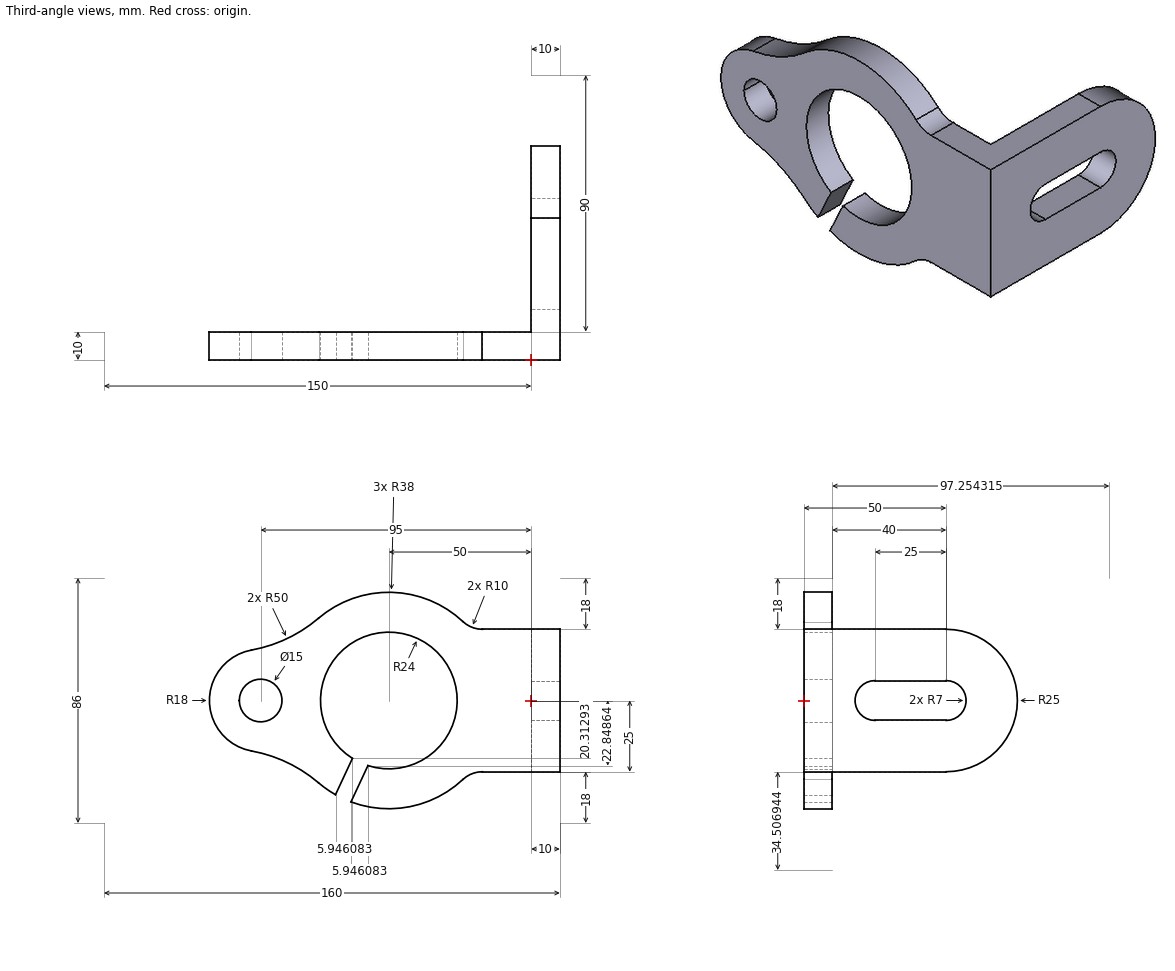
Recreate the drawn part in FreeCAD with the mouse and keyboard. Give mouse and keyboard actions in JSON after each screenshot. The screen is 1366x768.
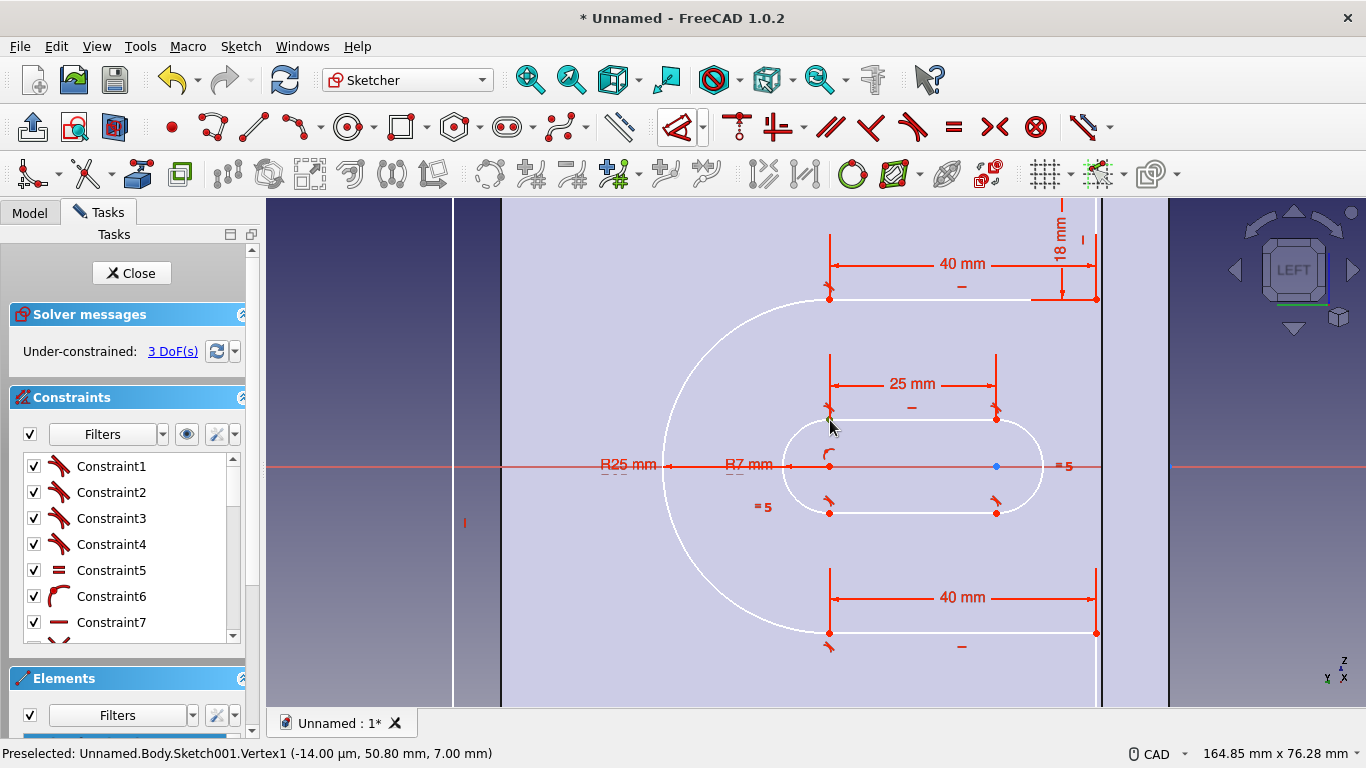
{"action": "key", "text": "l"}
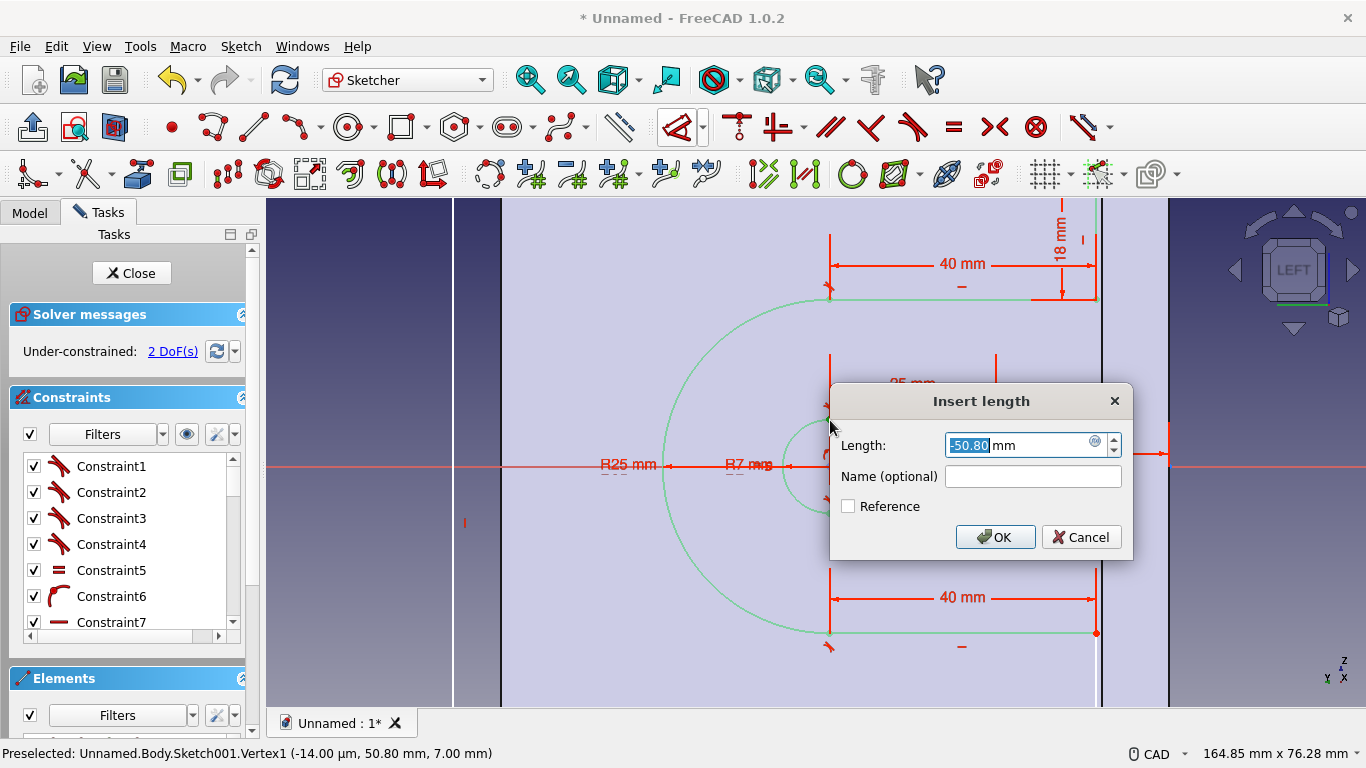
{"action": "type", "text": "-50"}
{"action": "key", "text": "Return"}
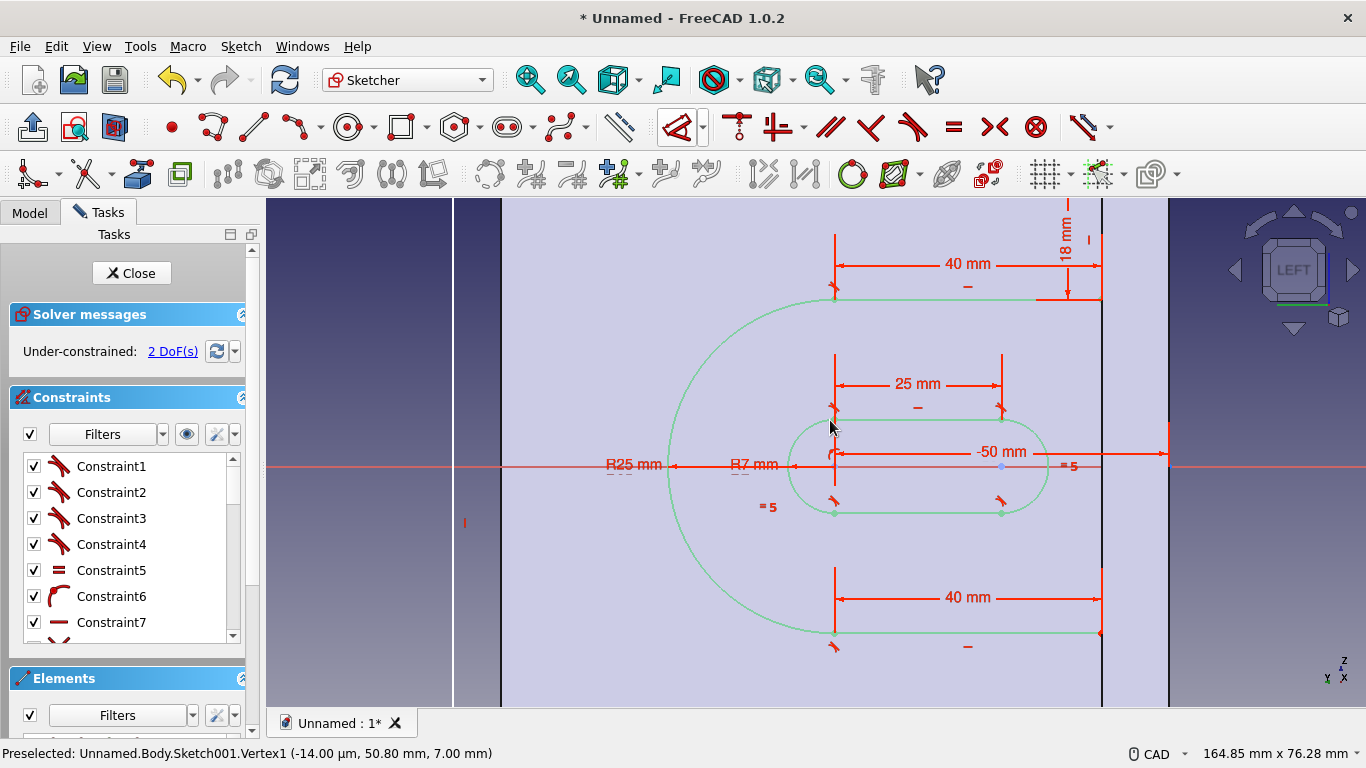
{"action": "scroll", "coordinate": [696, 396], "scroll_direction": "down", "scroll_amount": 4}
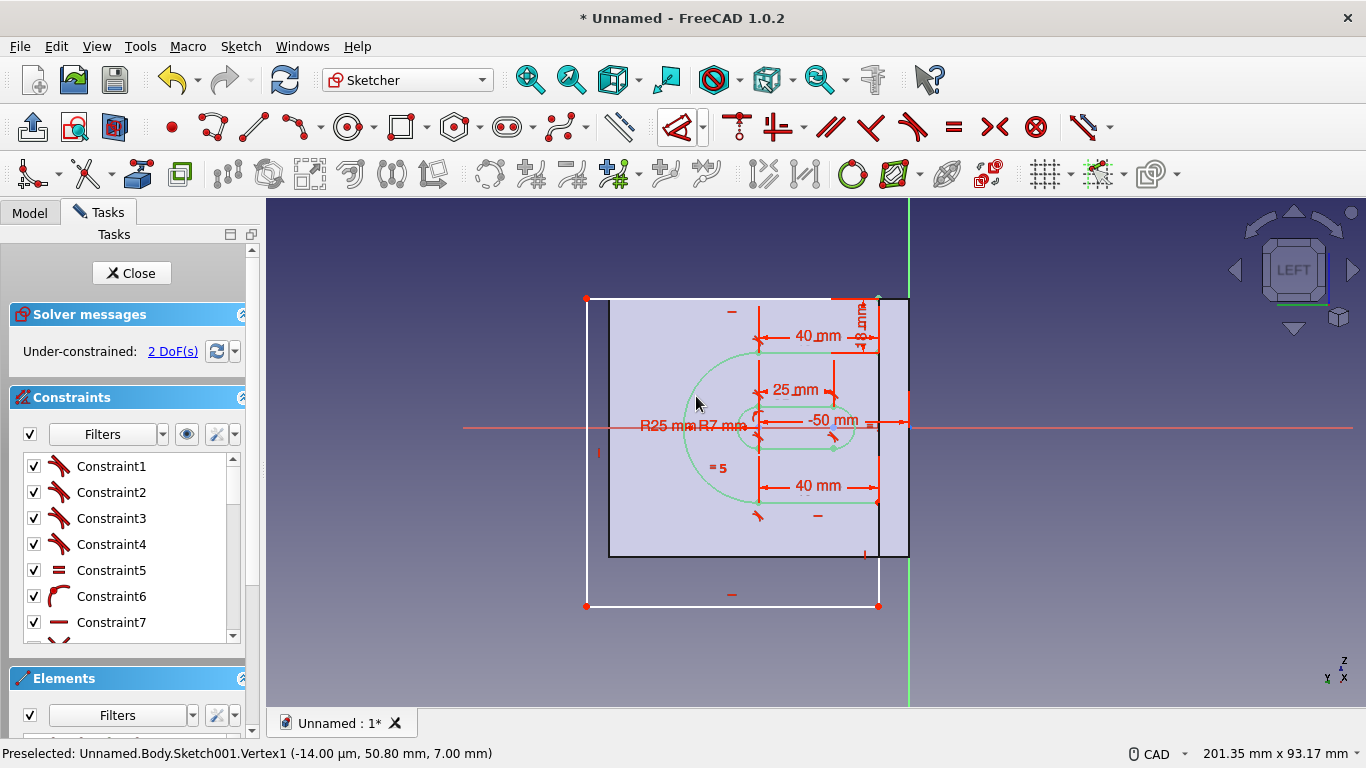
{"action": "left_click", "coordinate": [791, 299]}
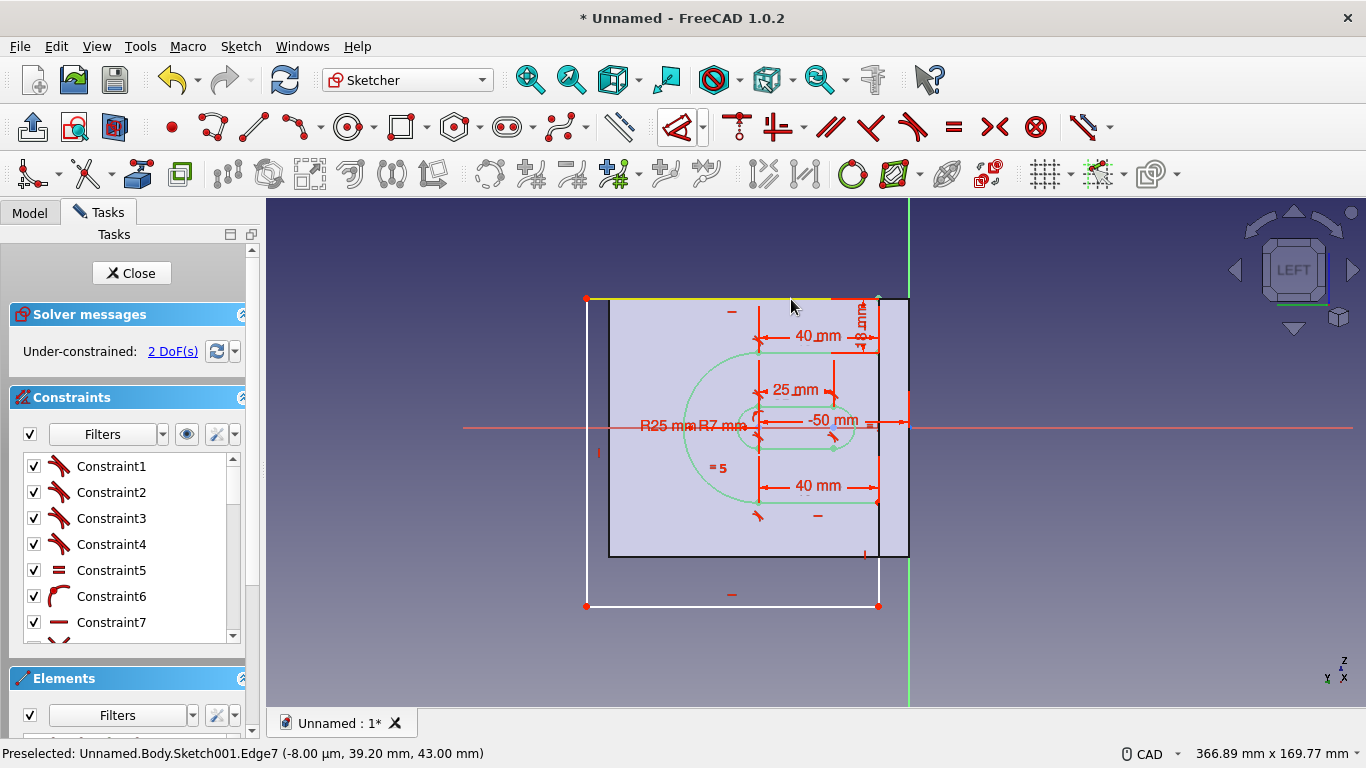
{"action": "left_click", "coordinate": [702, 128]}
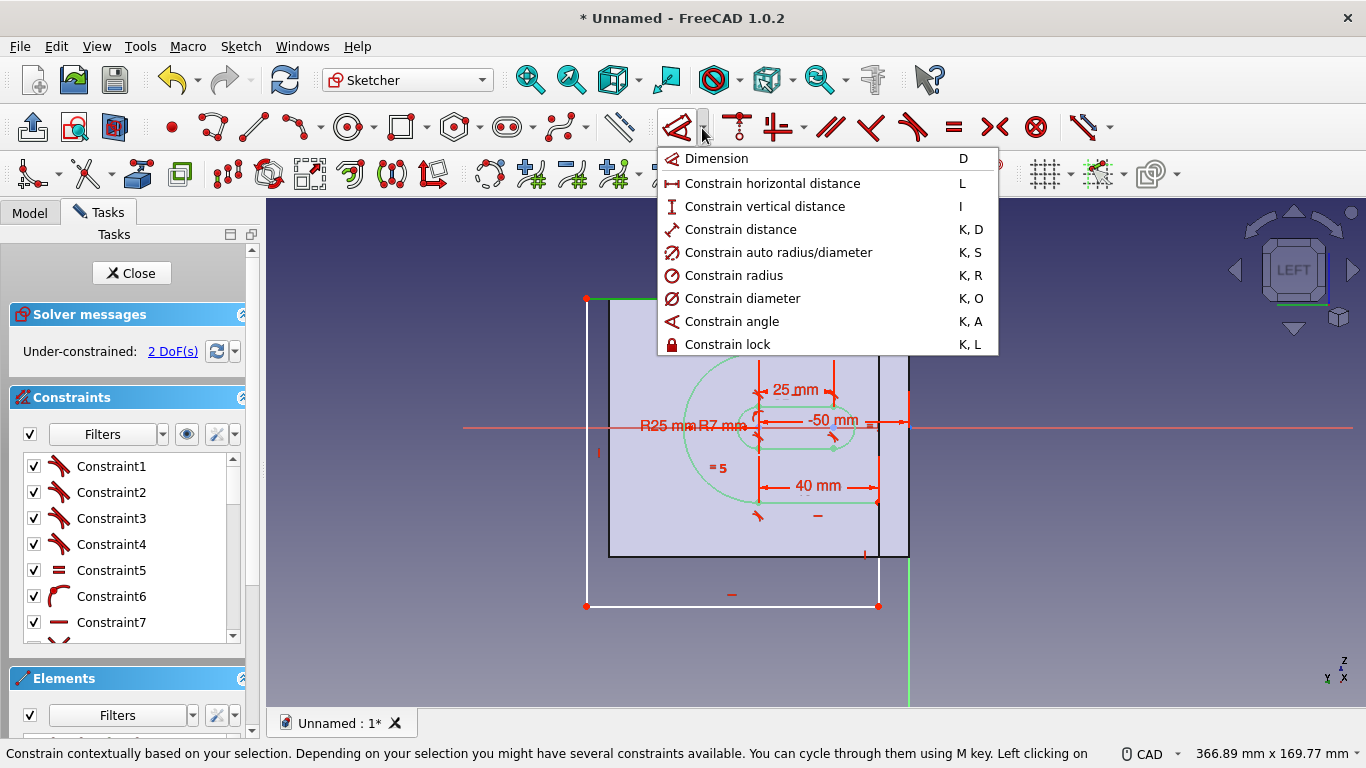
{"action": "left_click", "coordinate": [828, 184]}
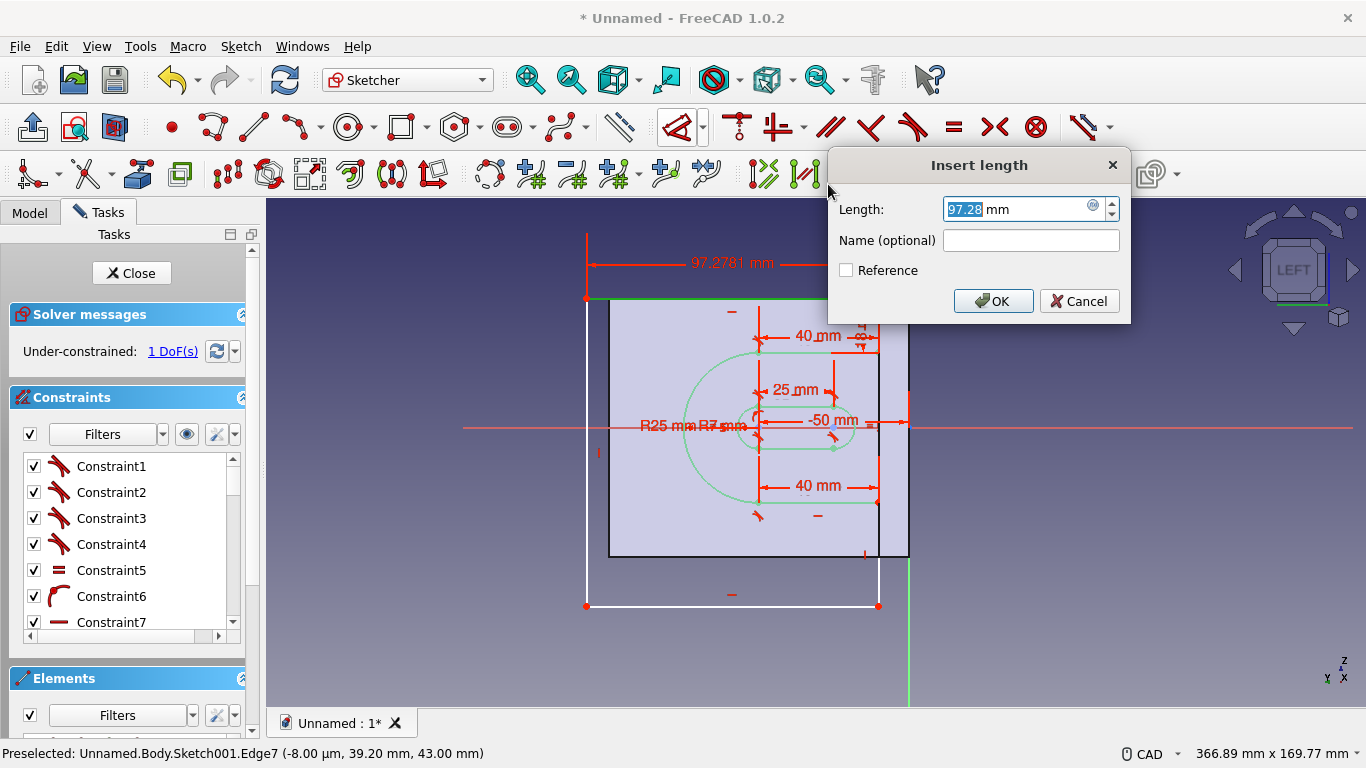
{"action": "type", "text": "97.254315"}
{"action": "key", "text": "Return"}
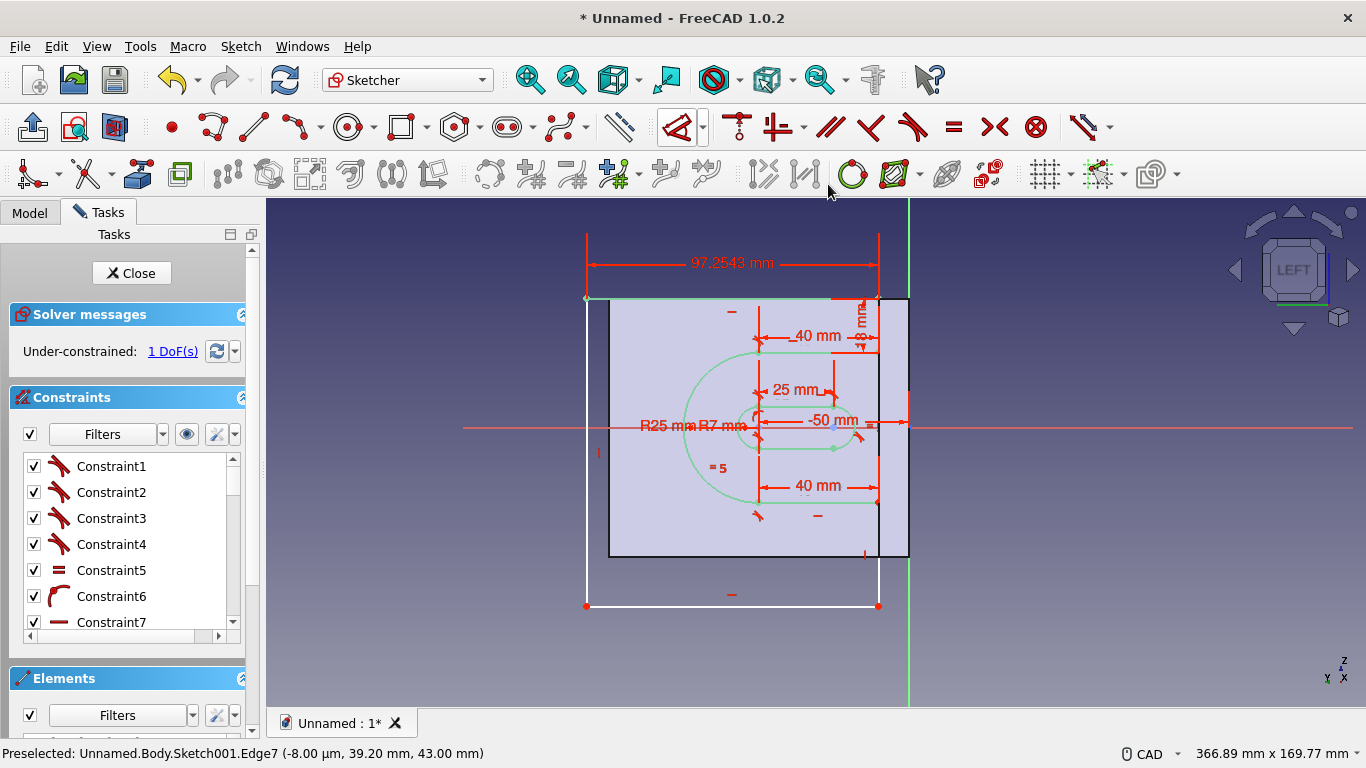
{"action": "left_click", "coordinate": [879, 576]}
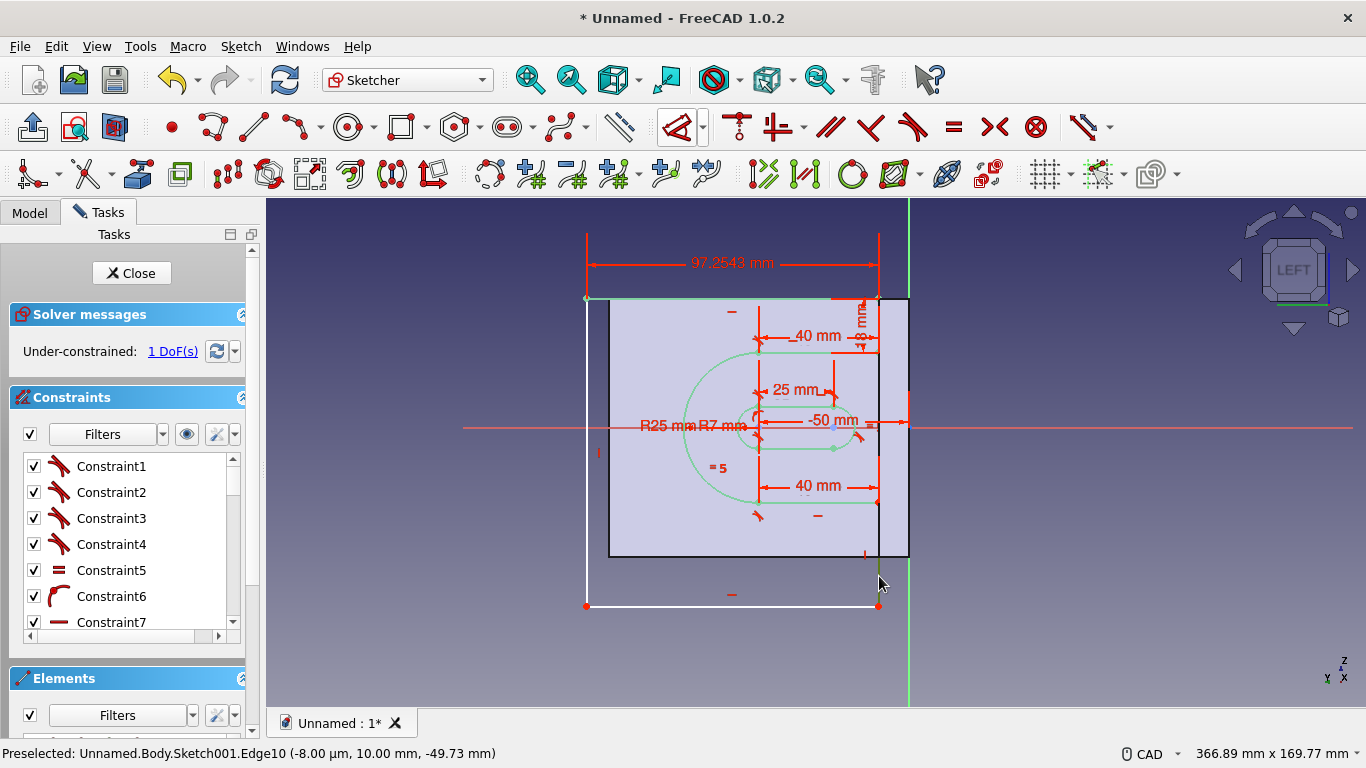
{"action": "key", "text": "i"}